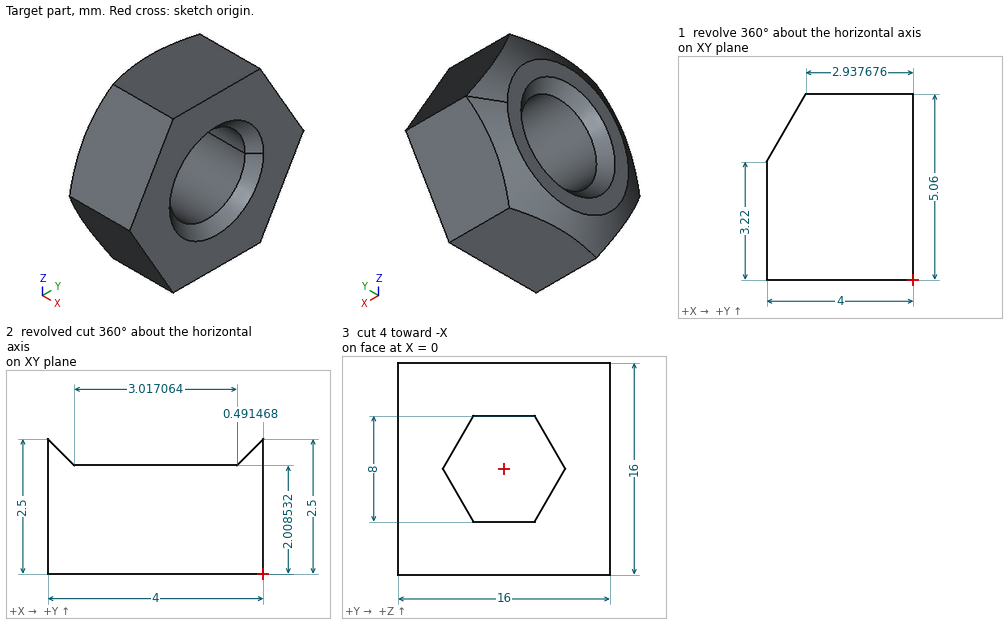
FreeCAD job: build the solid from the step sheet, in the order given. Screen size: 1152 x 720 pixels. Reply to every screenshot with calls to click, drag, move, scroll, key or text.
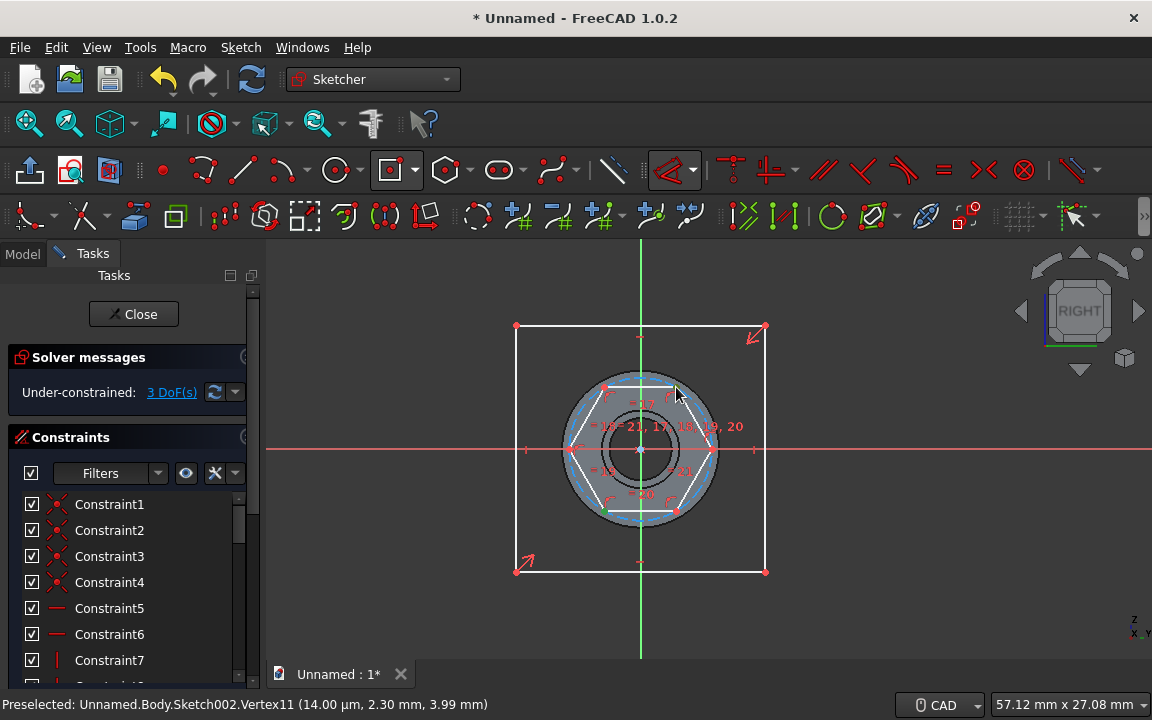
key(i)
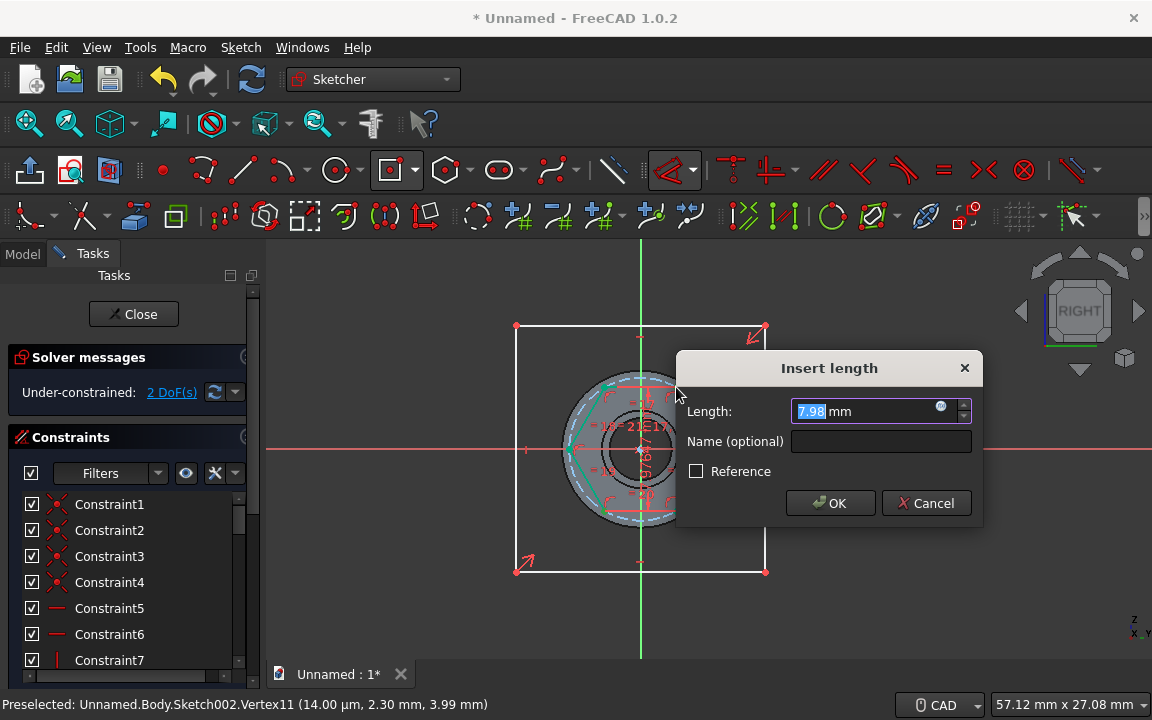
text(8)
key(Return)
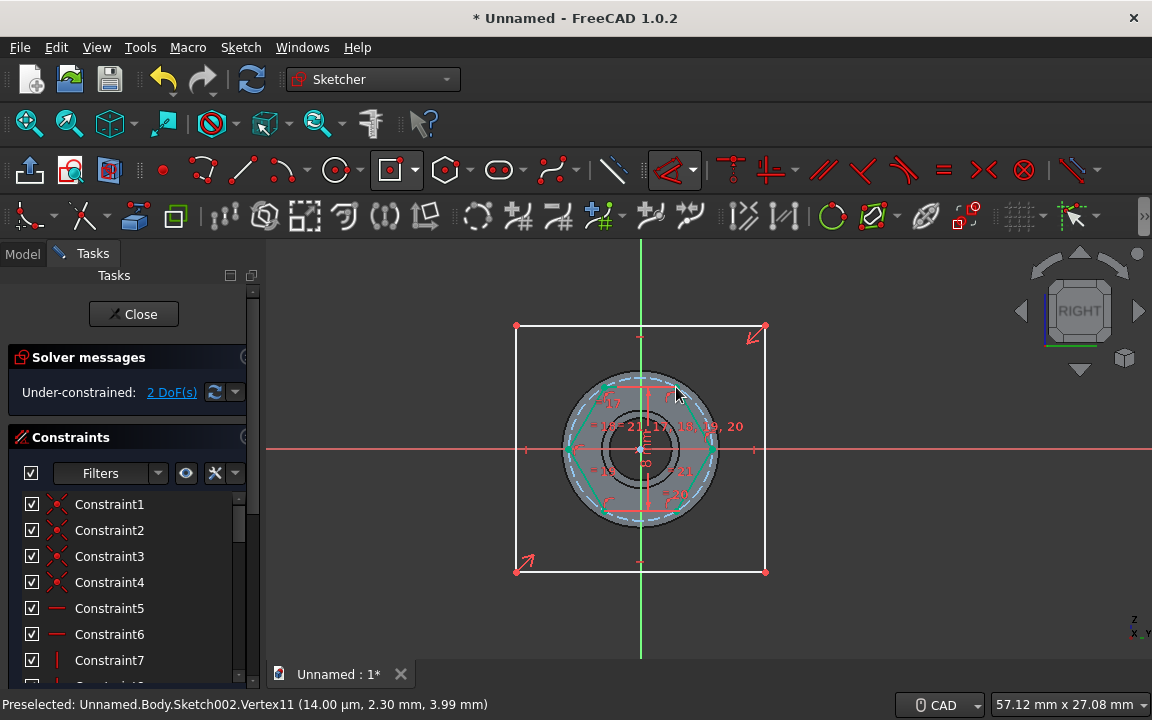
click(591, 572)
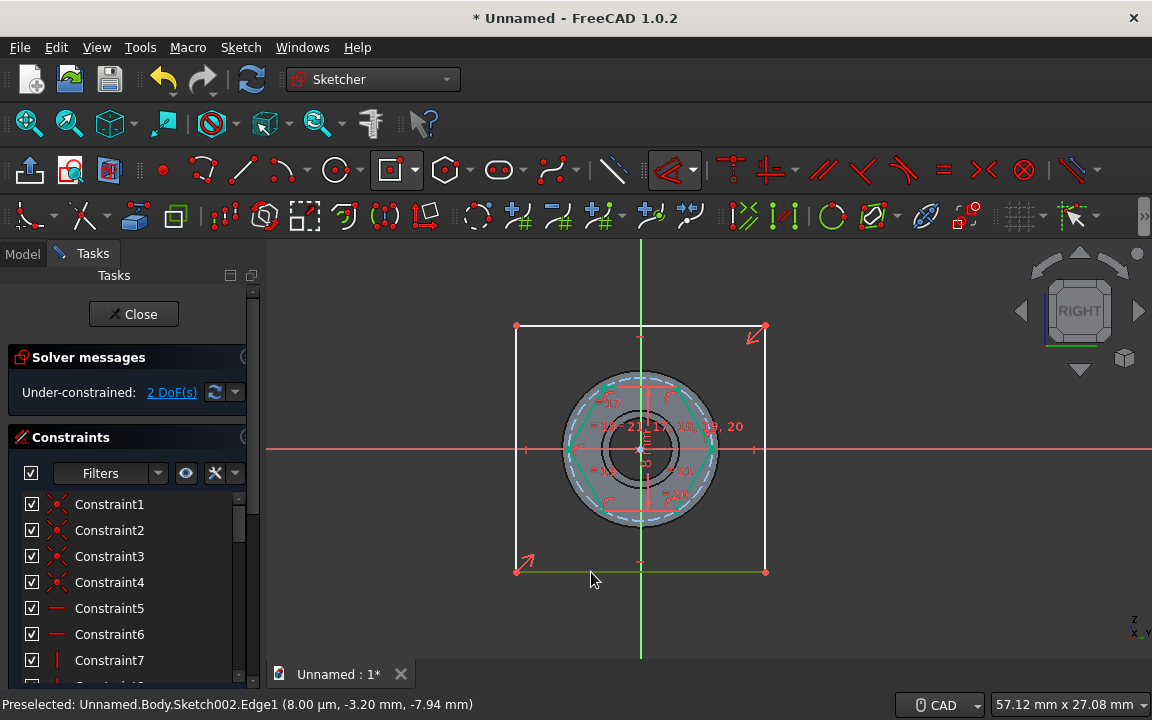
click(696, 170)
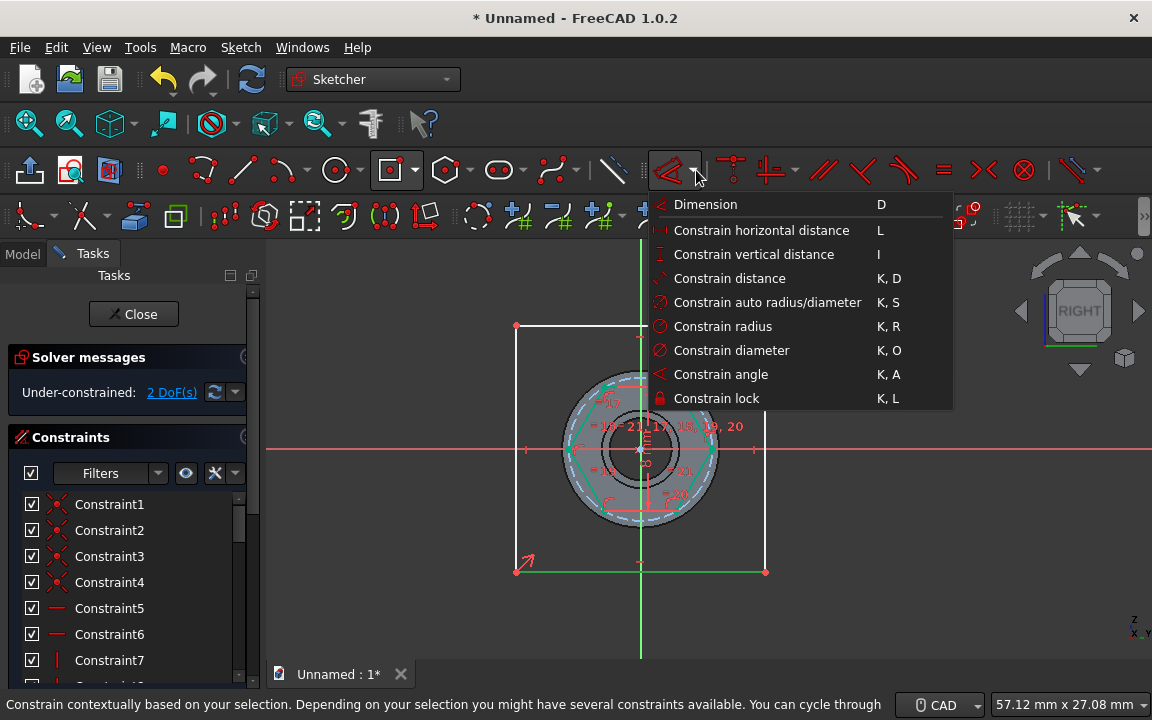
click(801, 230)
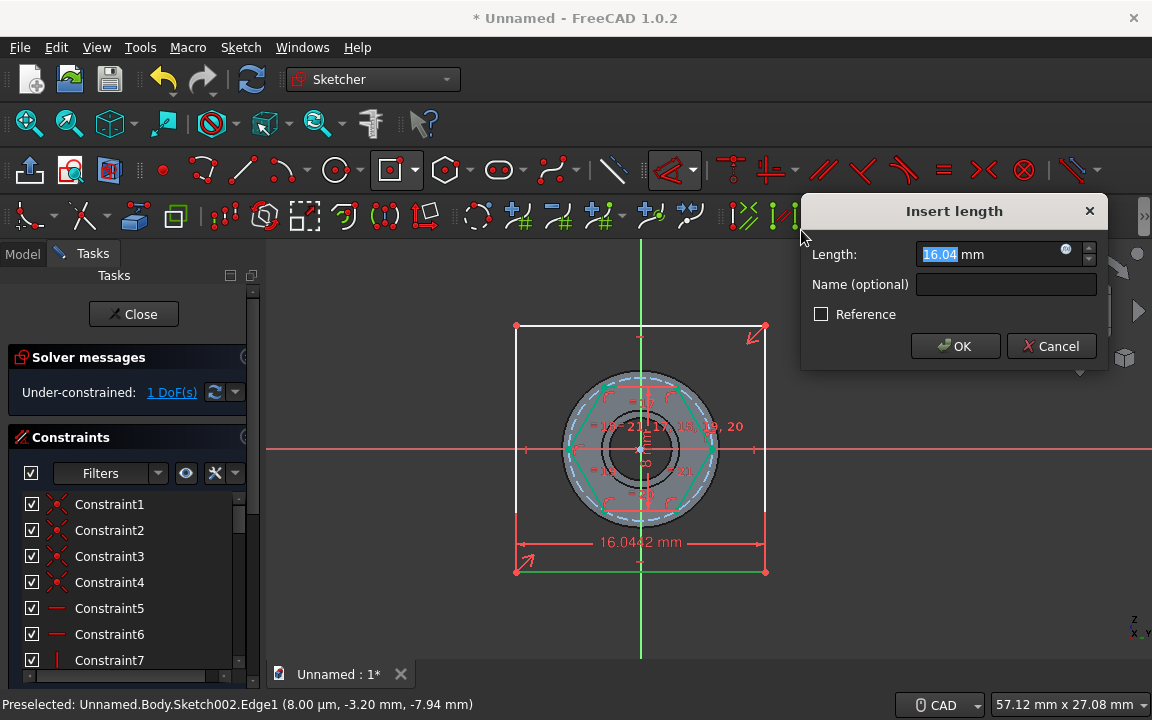
text(16)
key(Return)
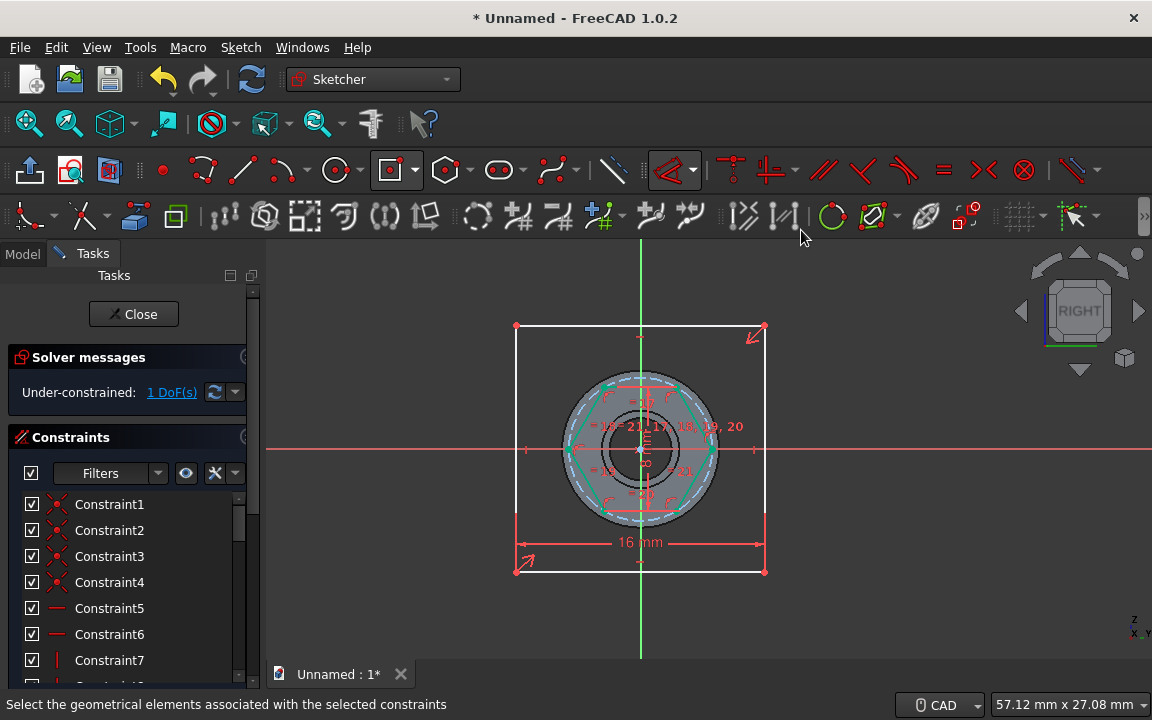
click(765, 499)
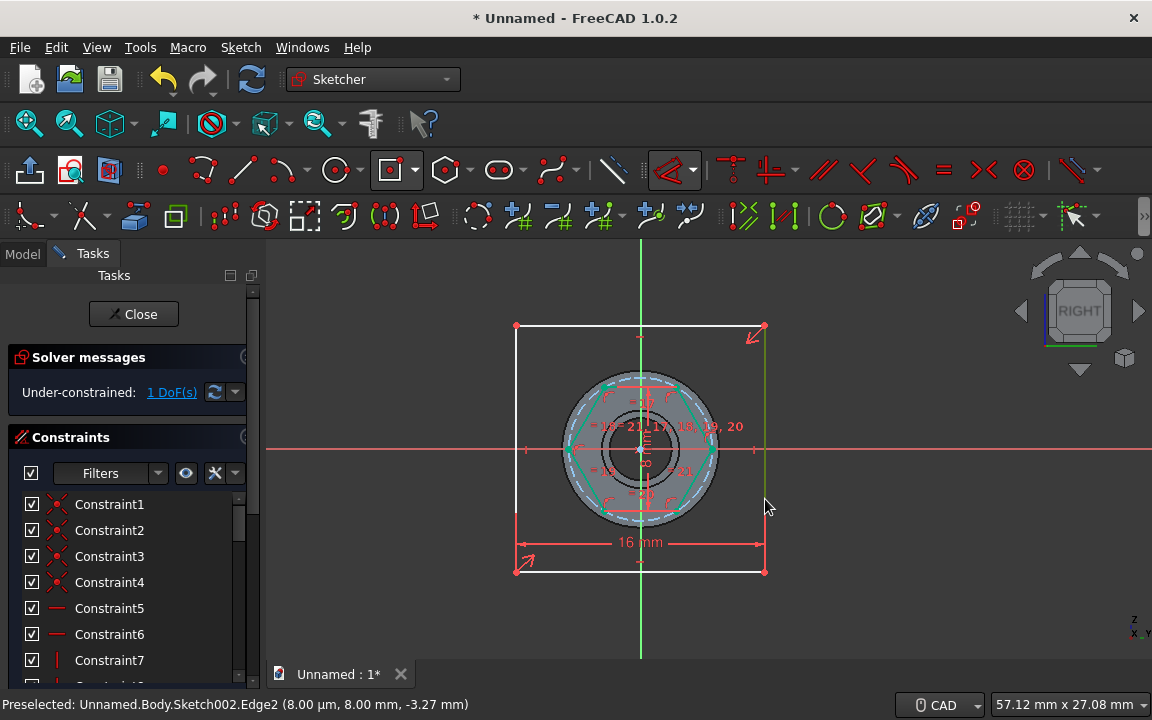
key(i)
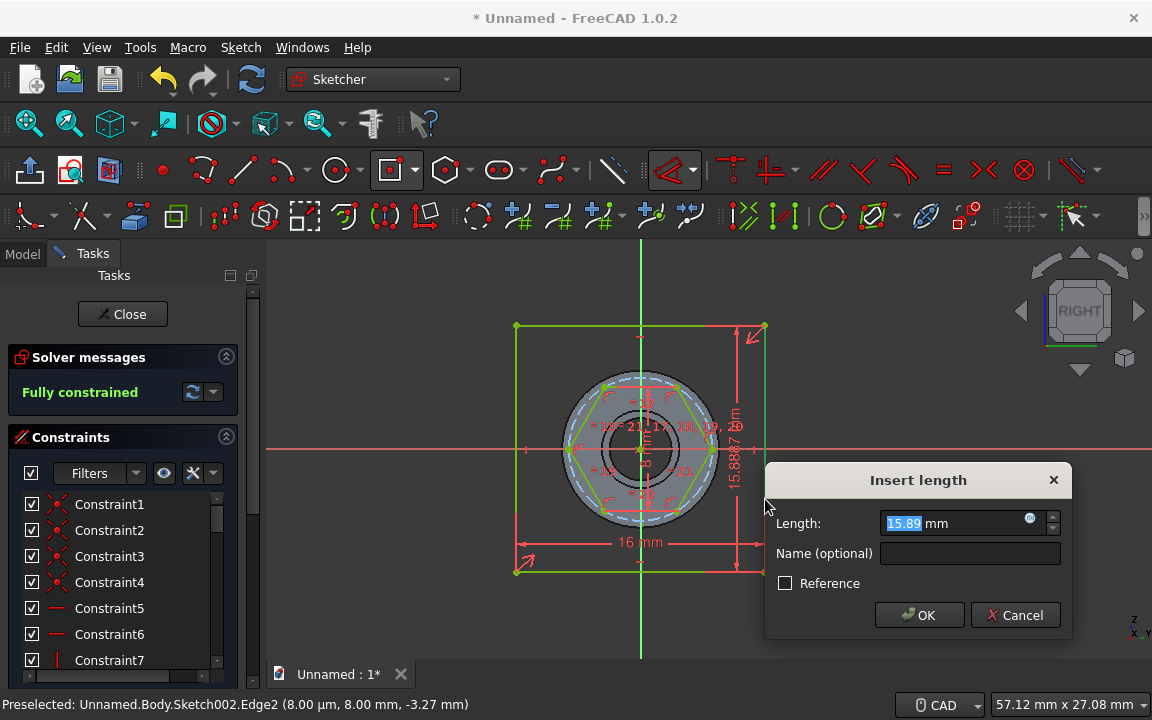
text(16)
key(Return)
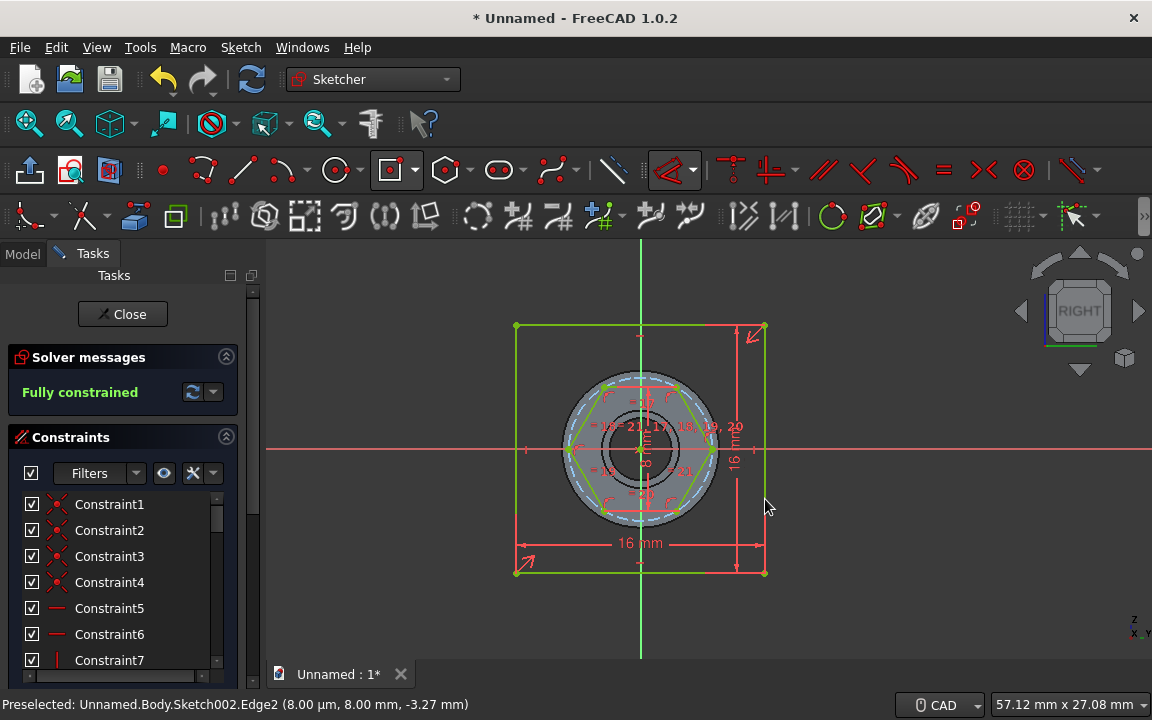
click(123, 314)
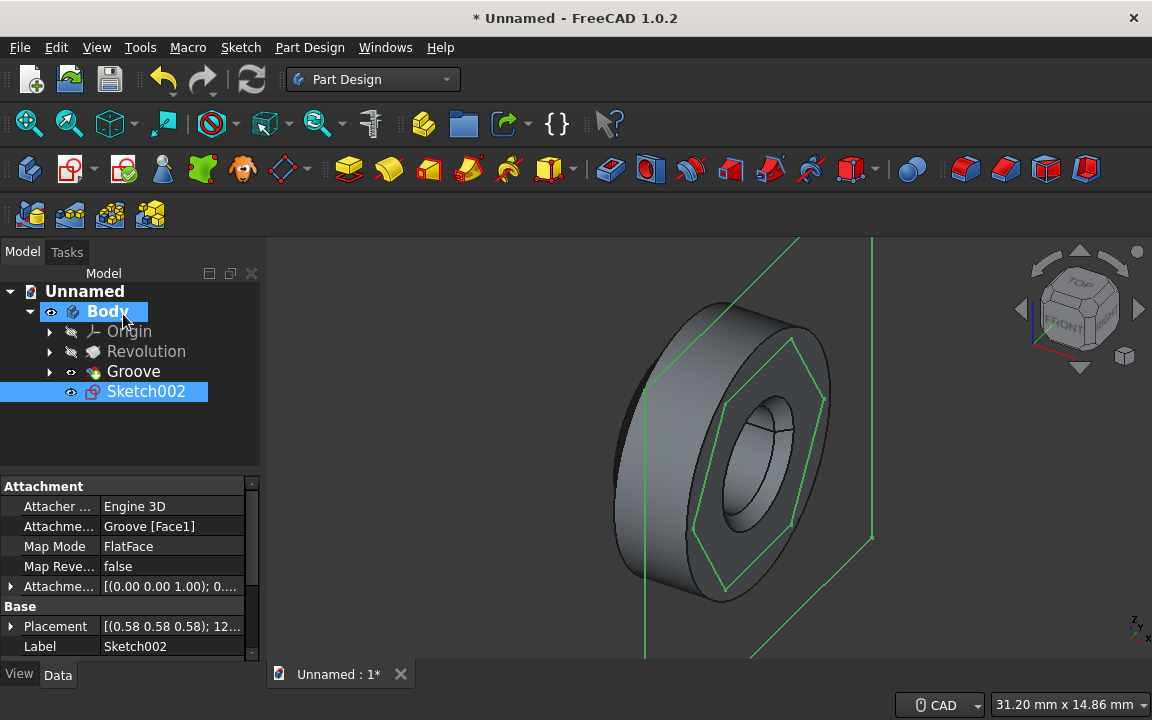
click(612, 170)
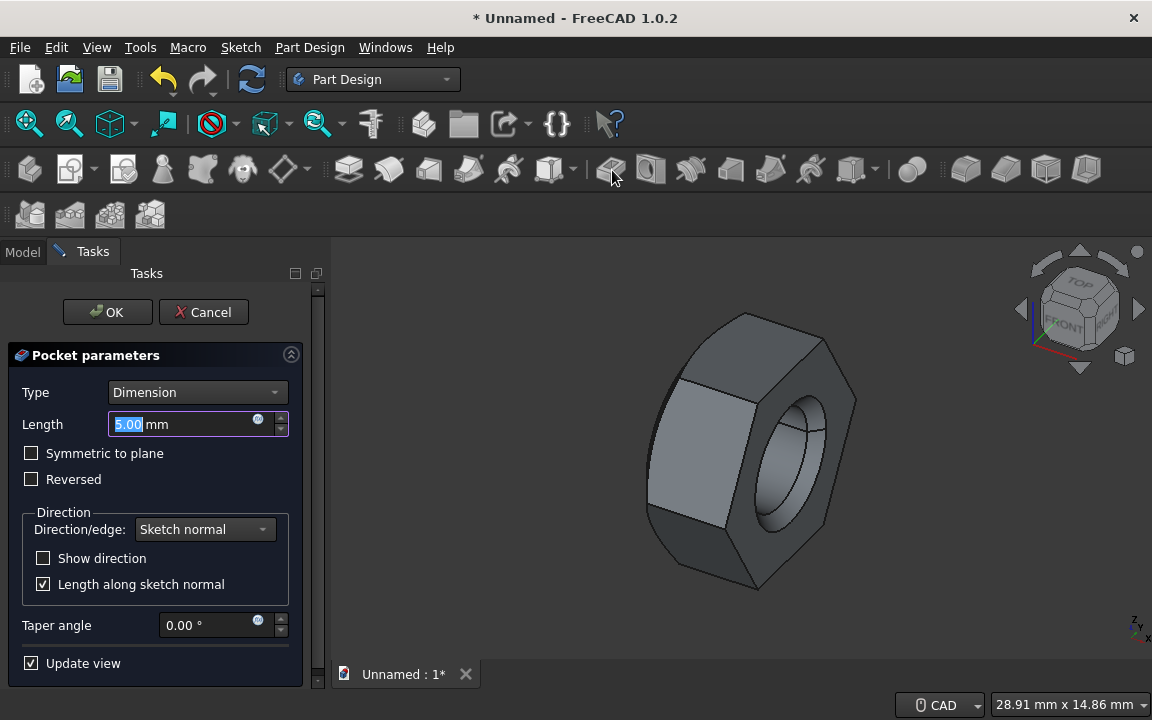
text(4)
key(Tab)